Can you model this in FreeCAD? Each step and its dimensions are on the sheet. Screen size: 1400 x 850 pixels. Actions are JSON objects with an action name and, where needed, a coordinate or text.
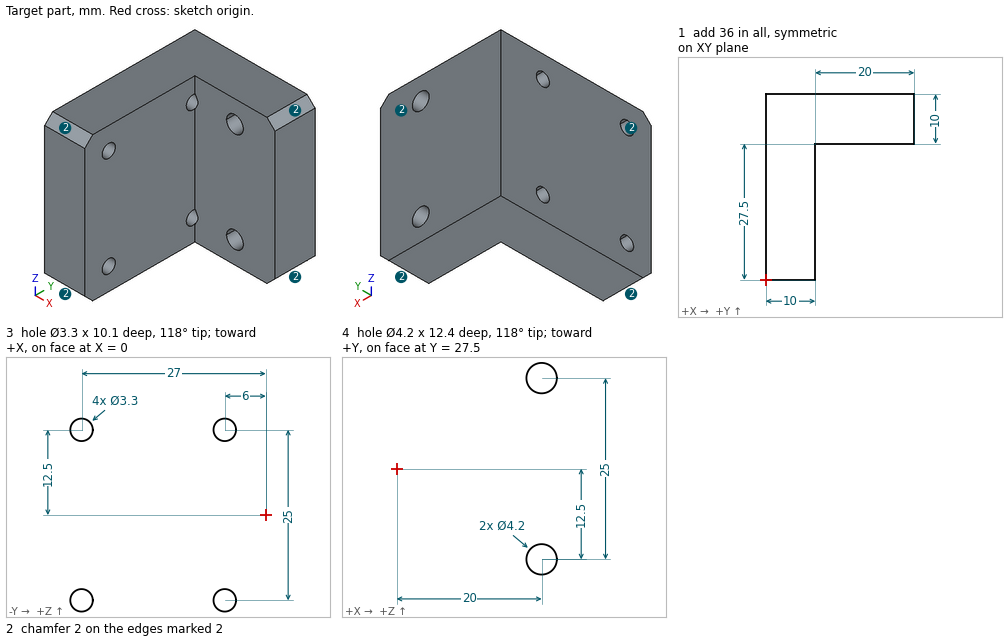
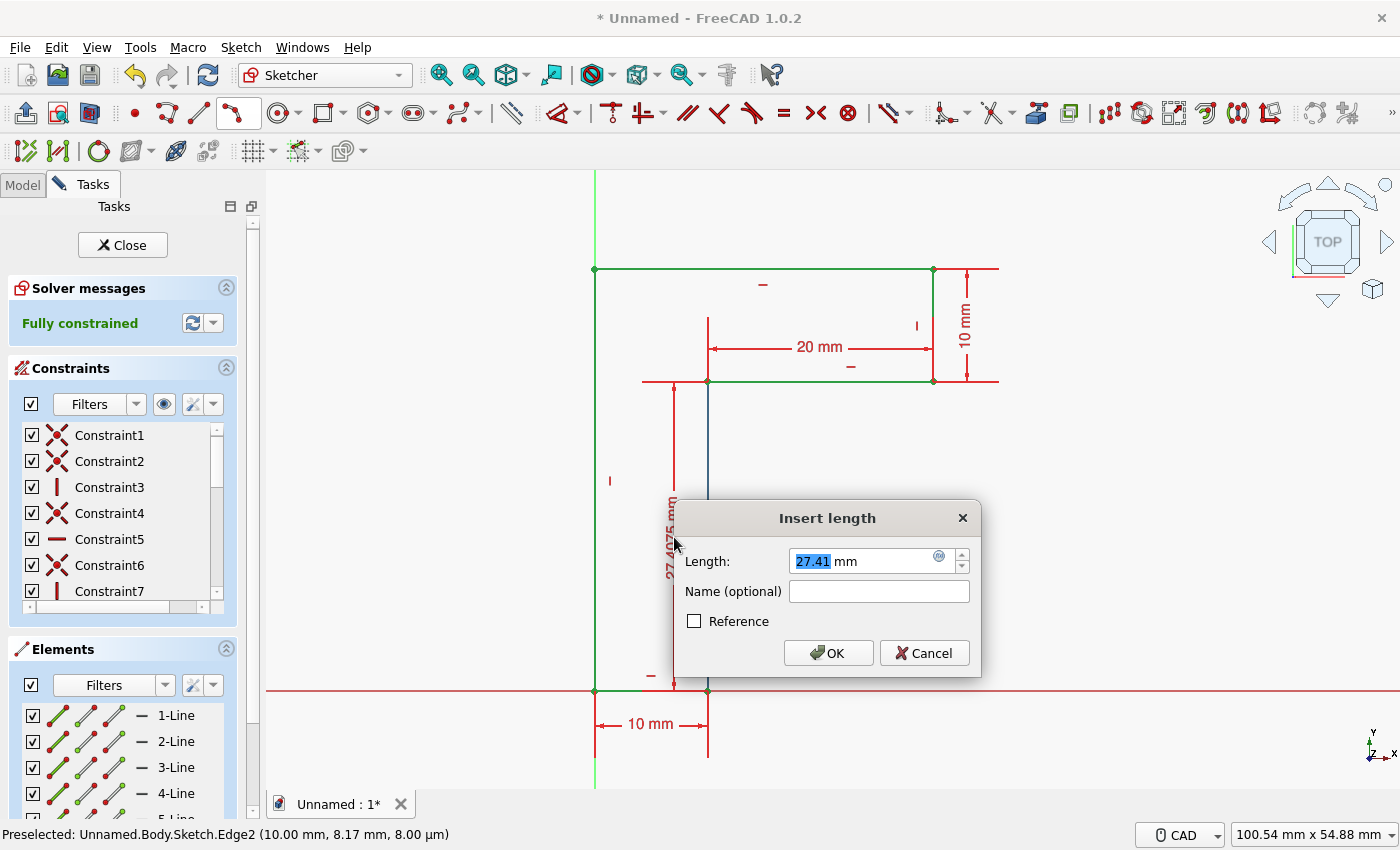
{"action": "type", "text": "27.5"}
{"action": "key", "text": "Return"}
{"action": "key", "text": "Escape"}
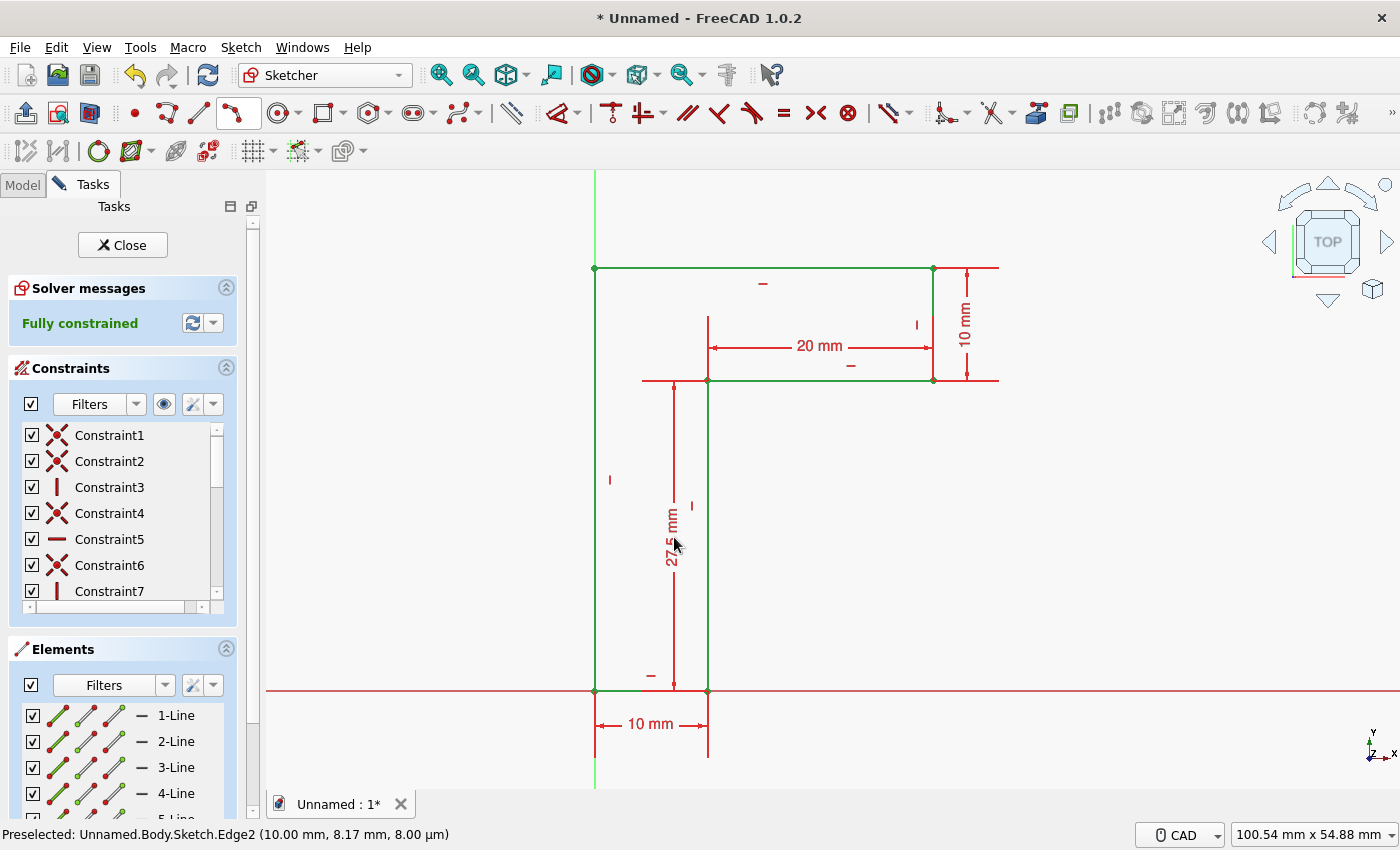
{"action": "left_click", "coordinate": [123, 245]}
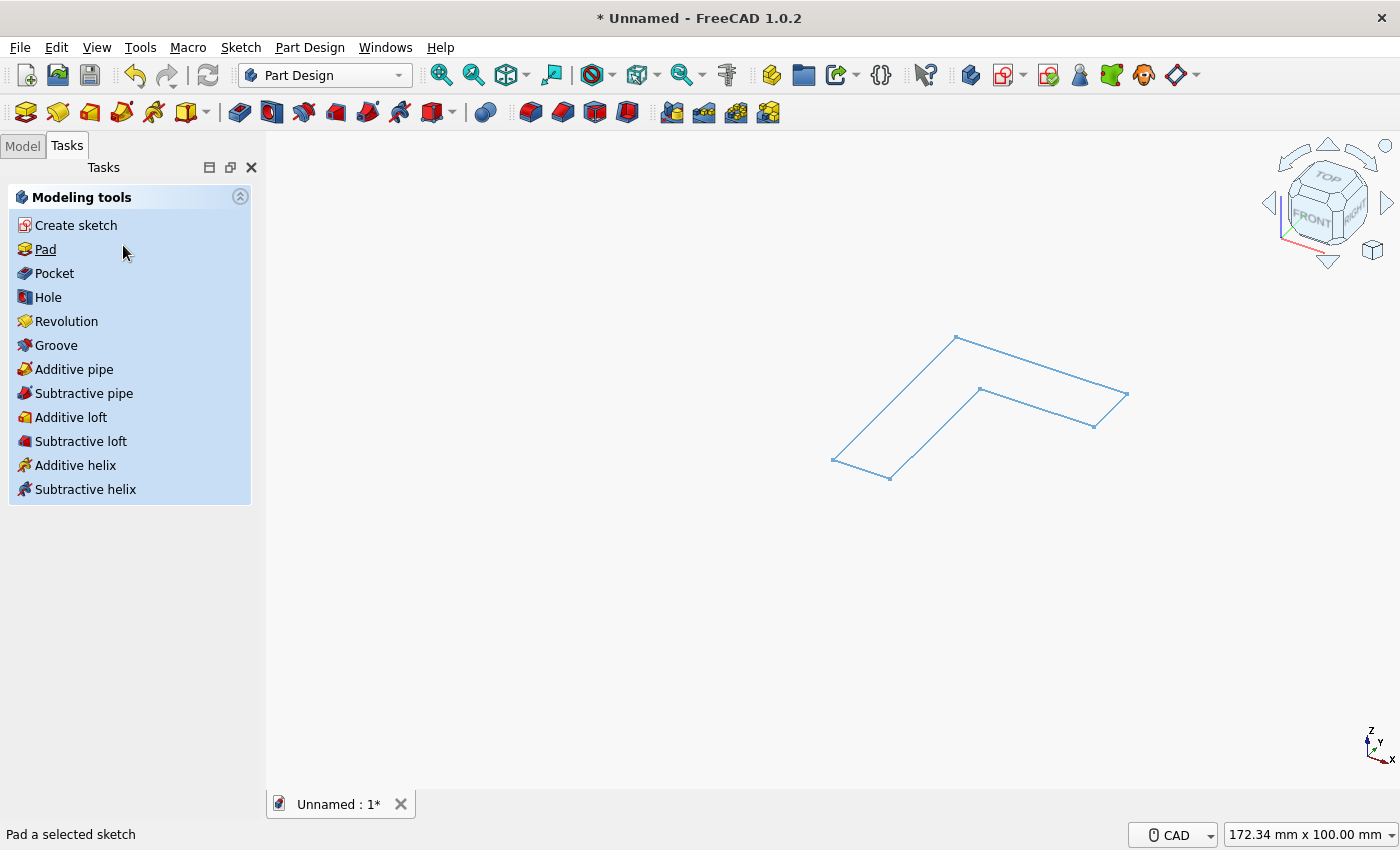
{"action": "left_click", "coordinate": [26, 112]}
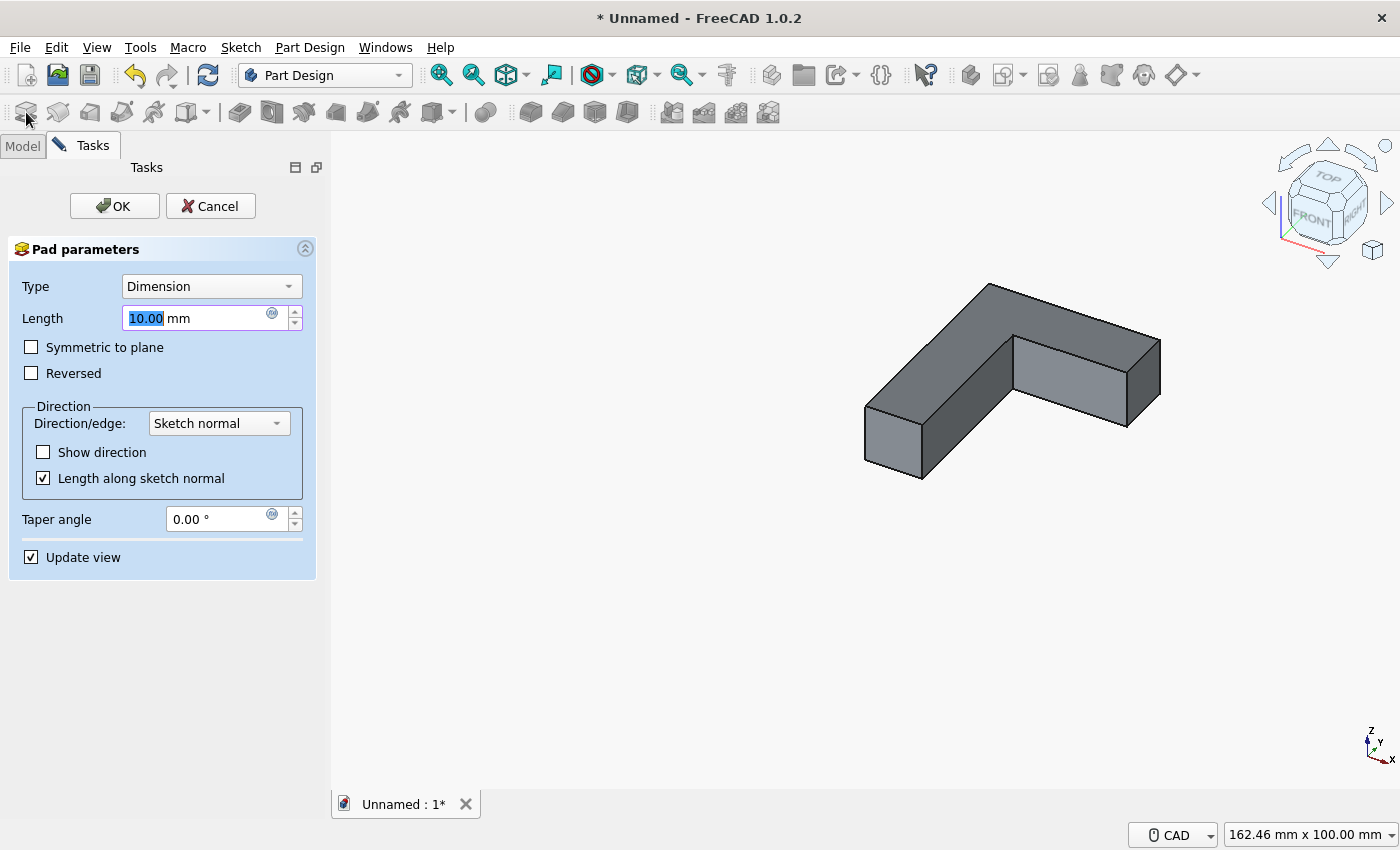
{"action": "type", "text": "36"}
{"action": "key", "text": "Tab"}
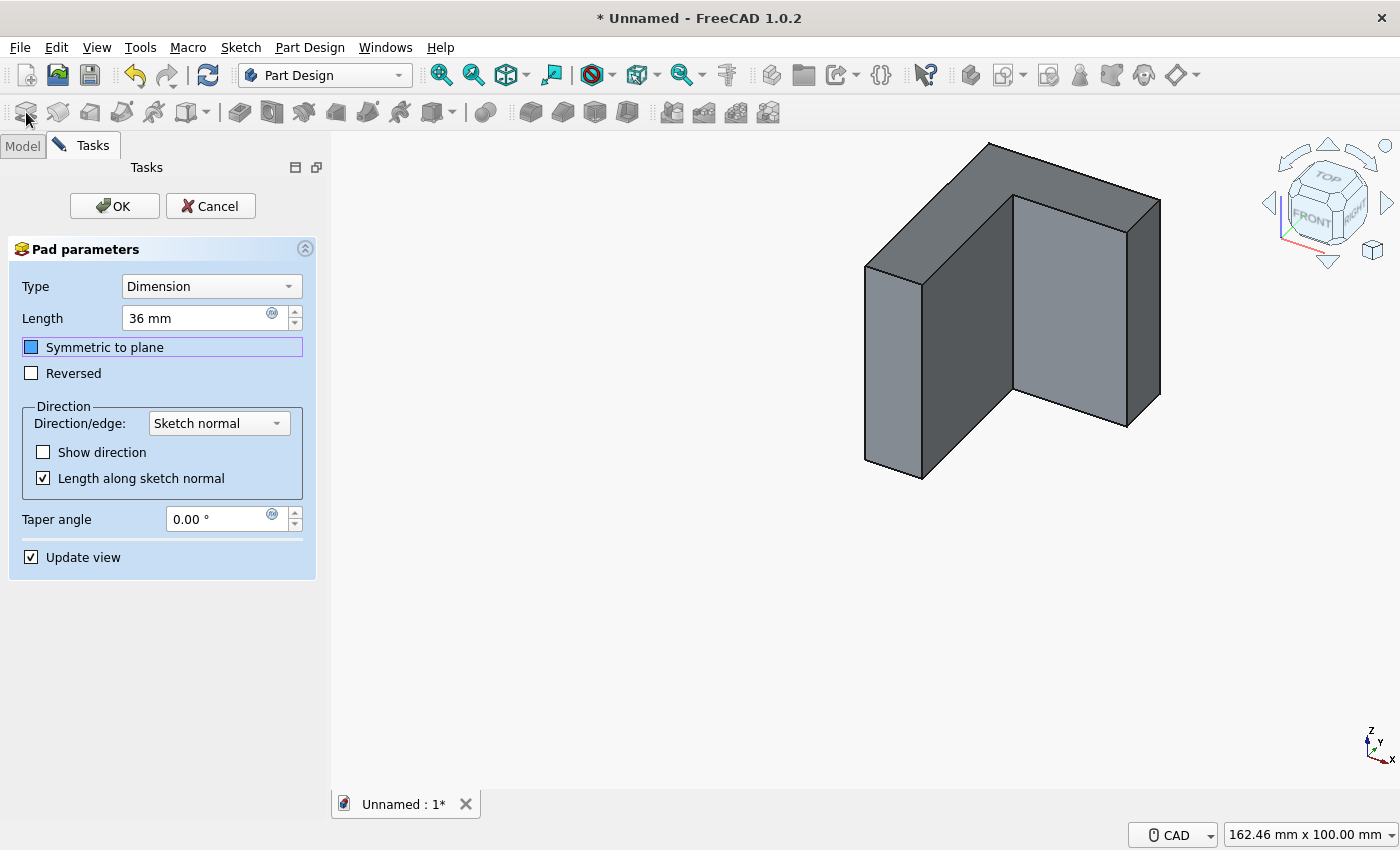
{"action": "left_click", "coordinate": [30, 347]}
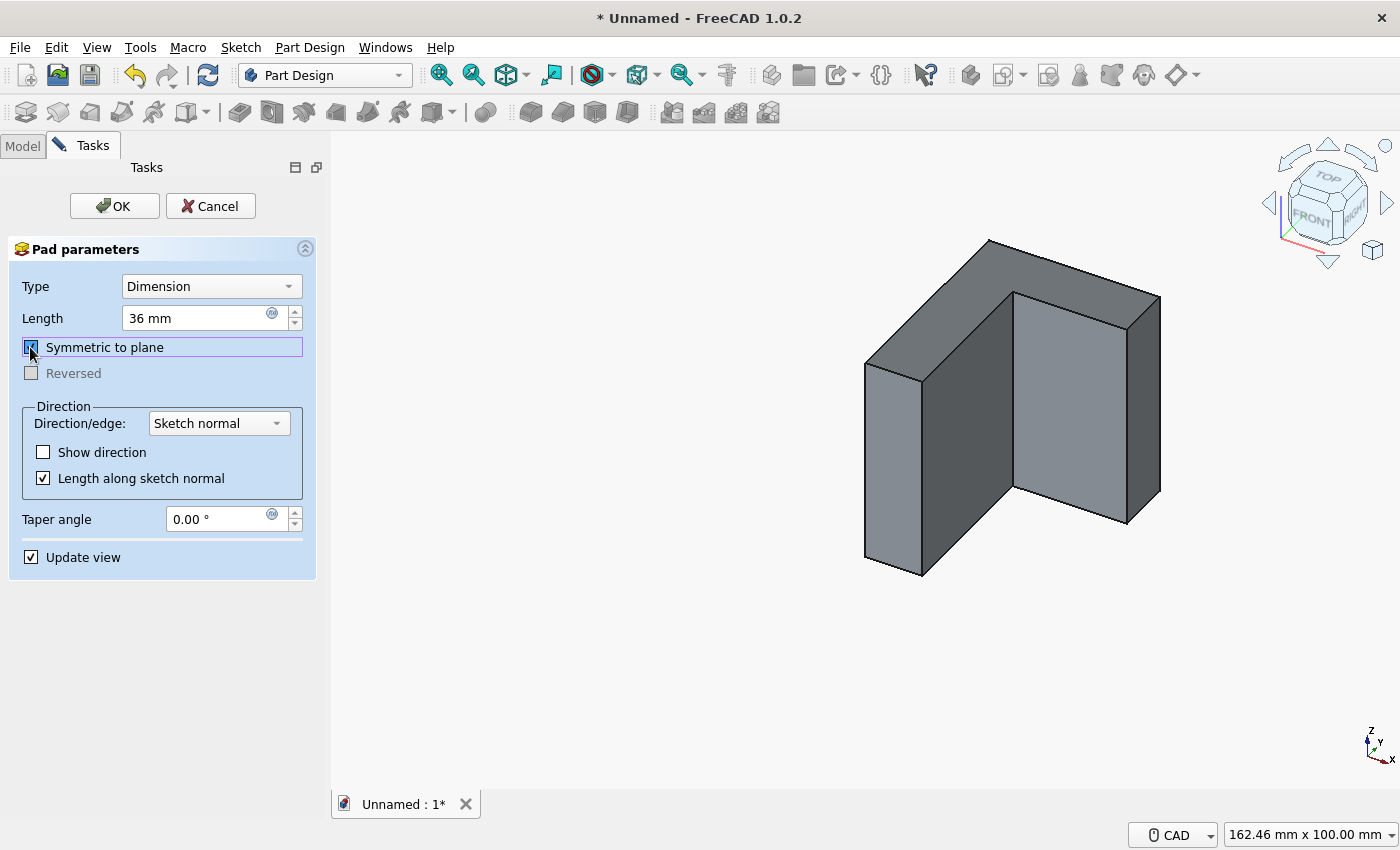
{"action": "left_click", "coordinate": [115, 206]}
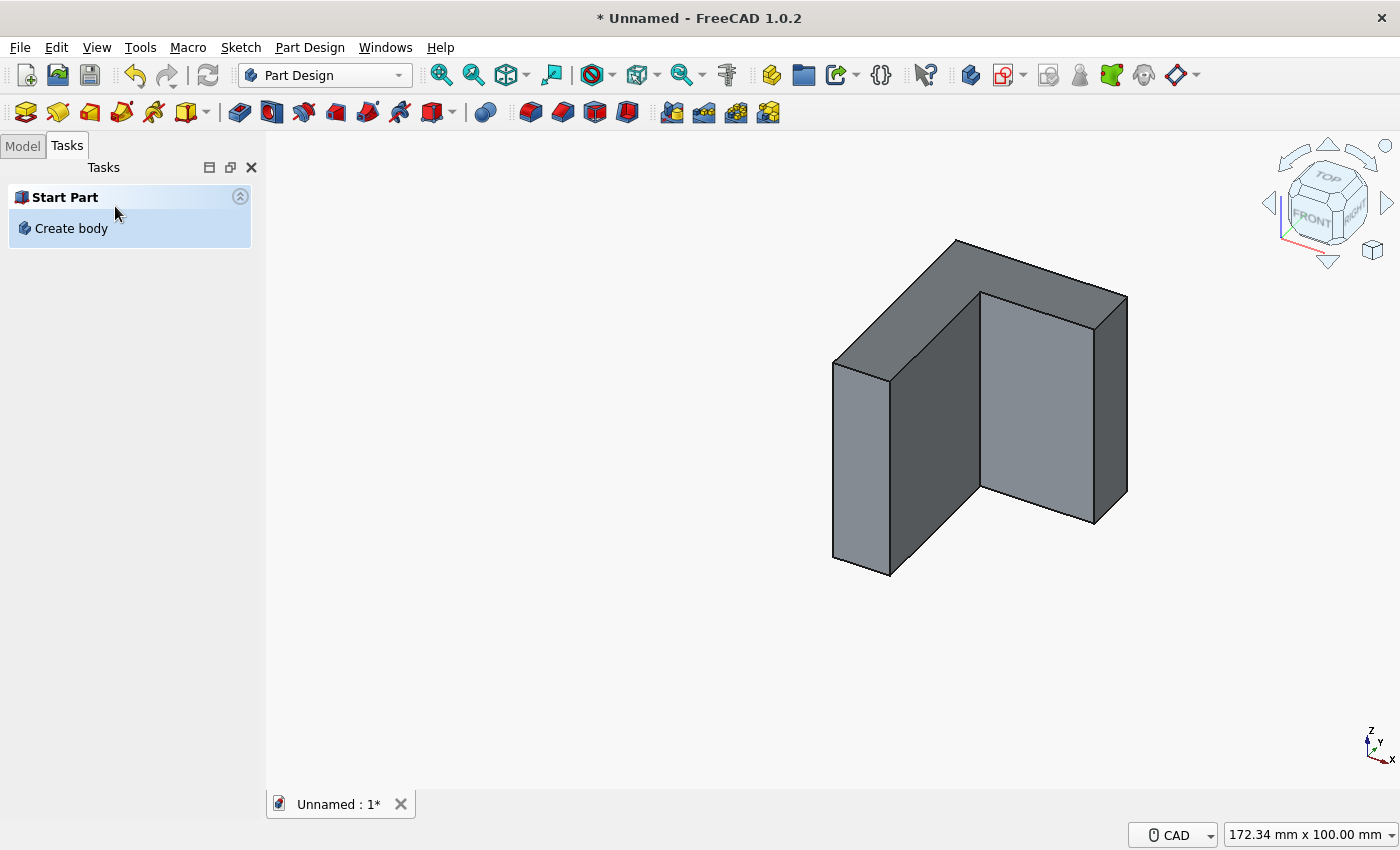
{"action": "left_click", "coordinate": [861, 371]}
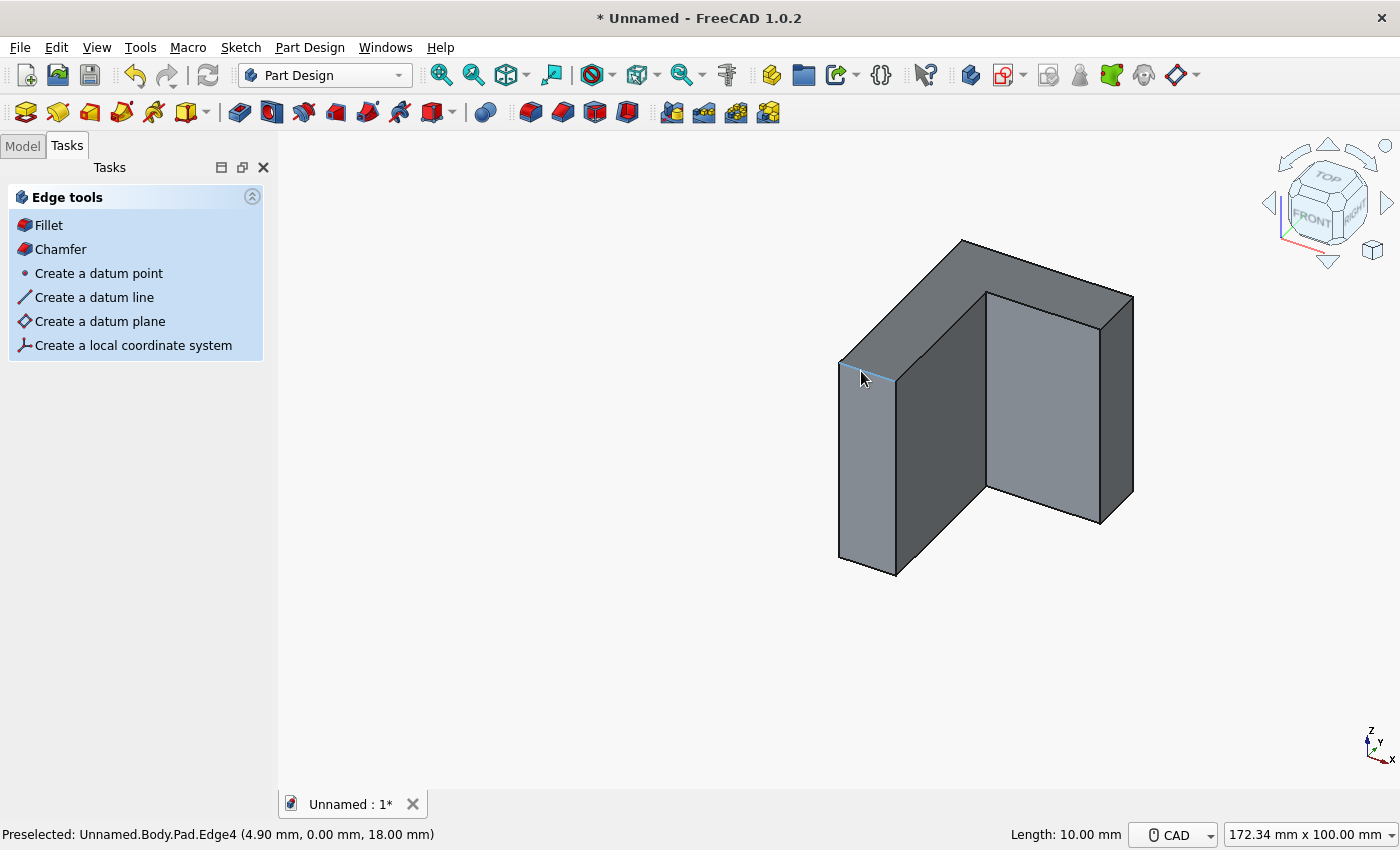
{"action": "left_click", "coordinate": [1117, 312], "text": "ctrl"}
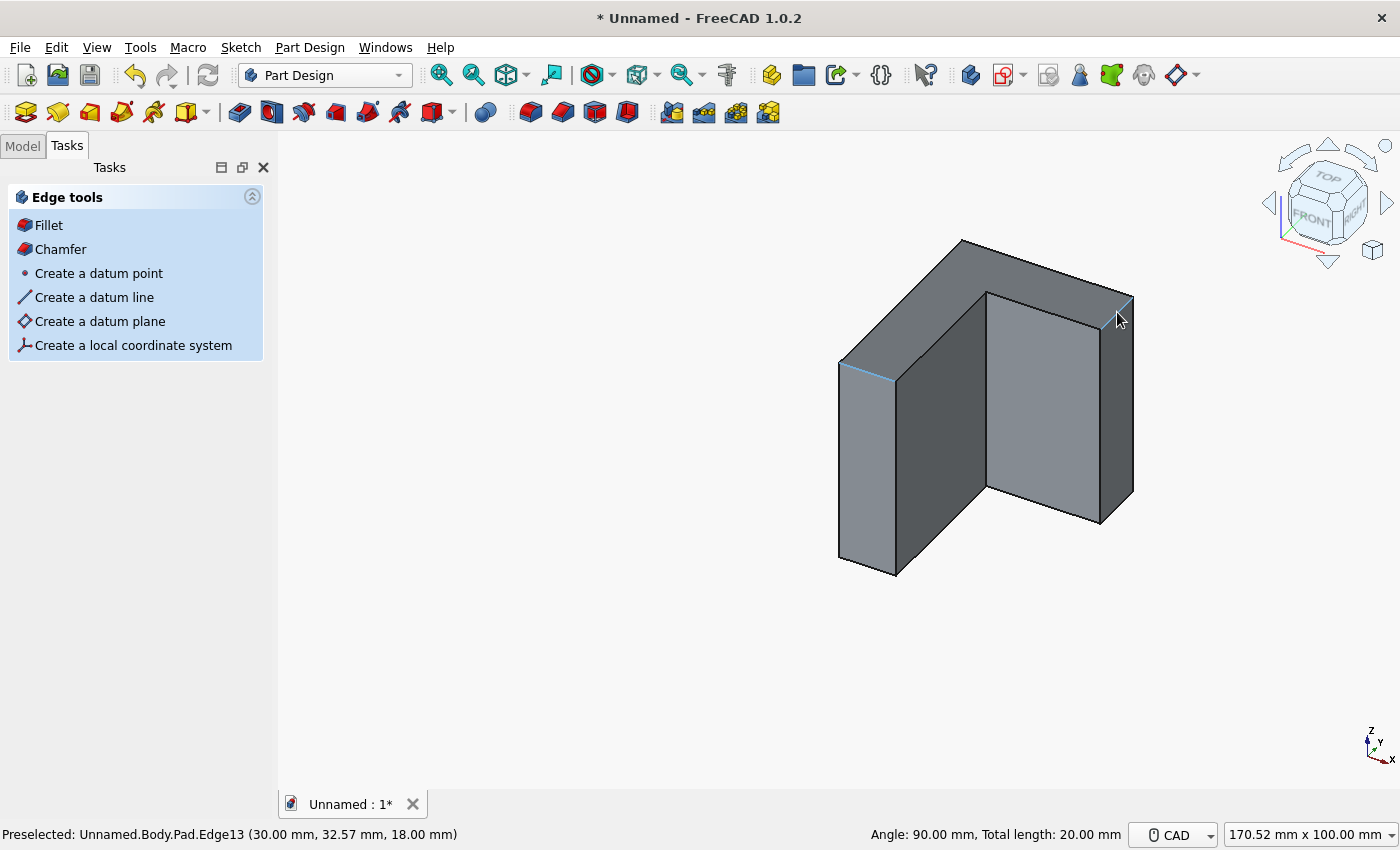
{"action": "key", "text": "0"}